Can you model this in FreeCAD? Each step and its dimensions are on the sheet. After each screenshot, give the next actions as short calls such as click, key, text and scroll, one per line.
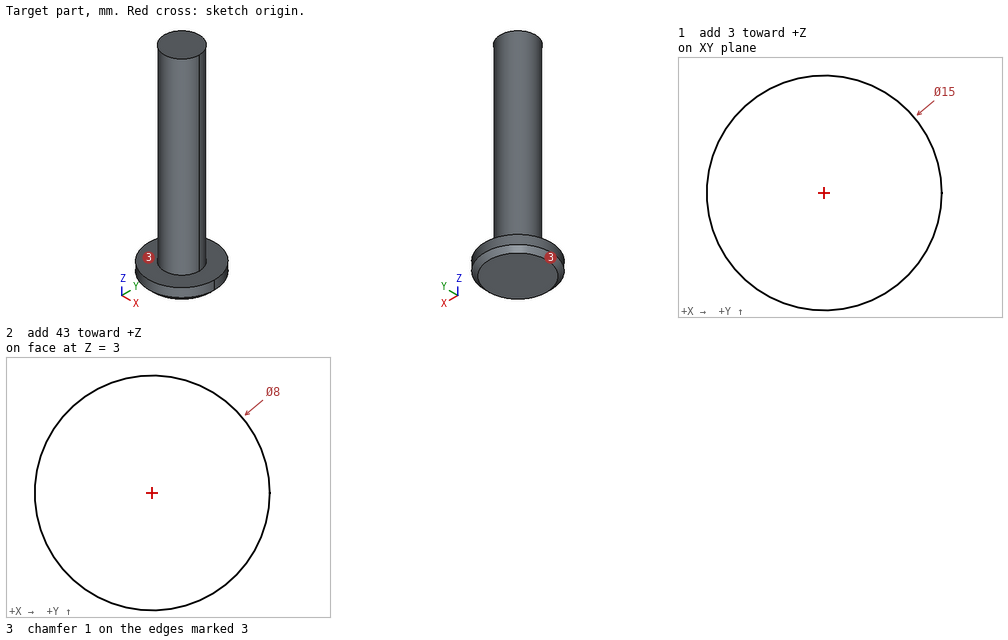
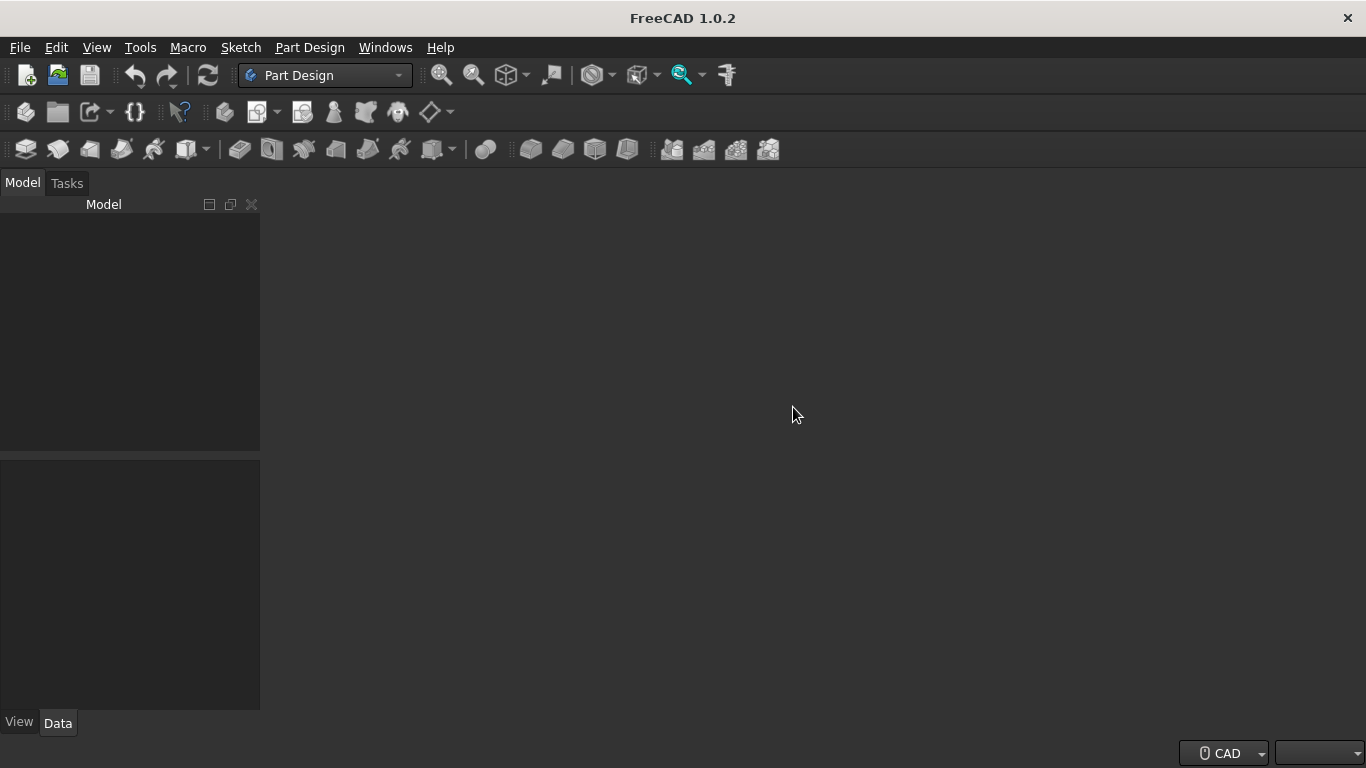
click(26, 76)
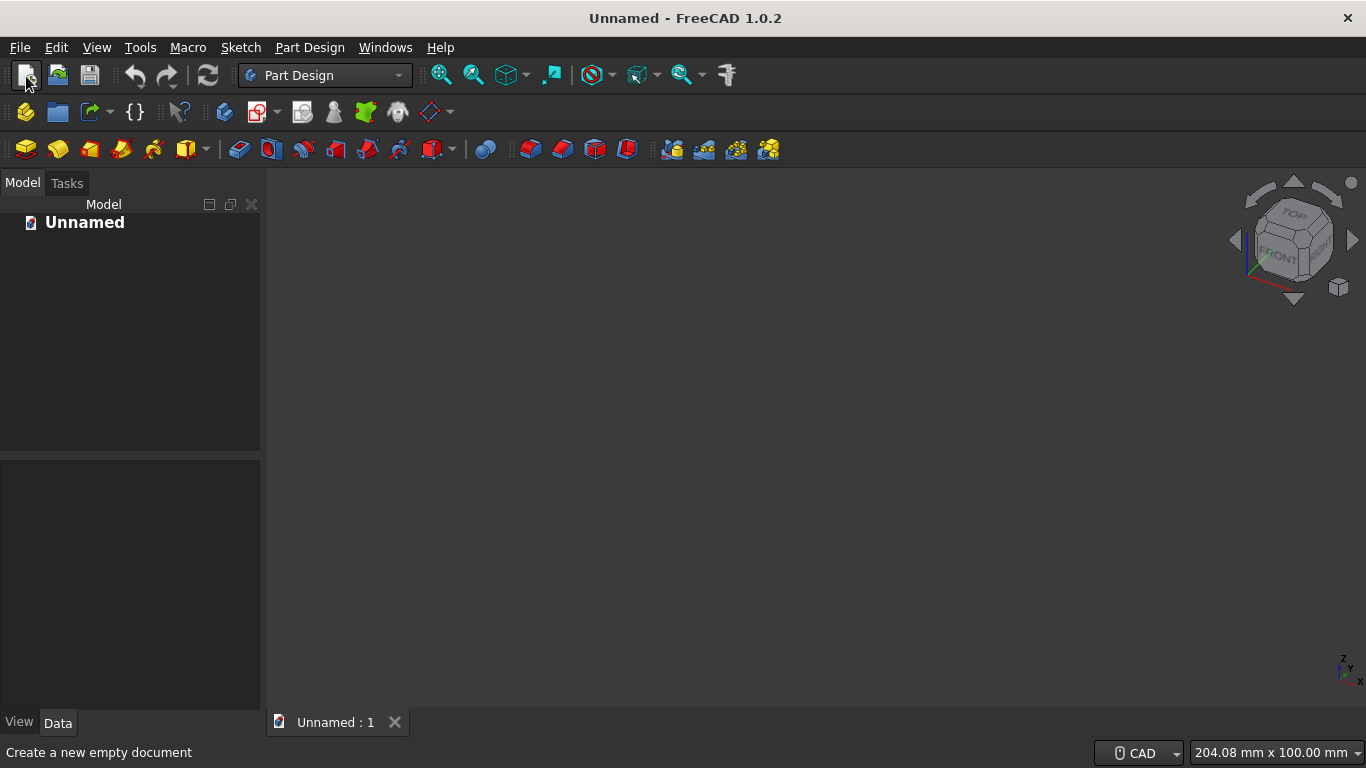
click(258, 112)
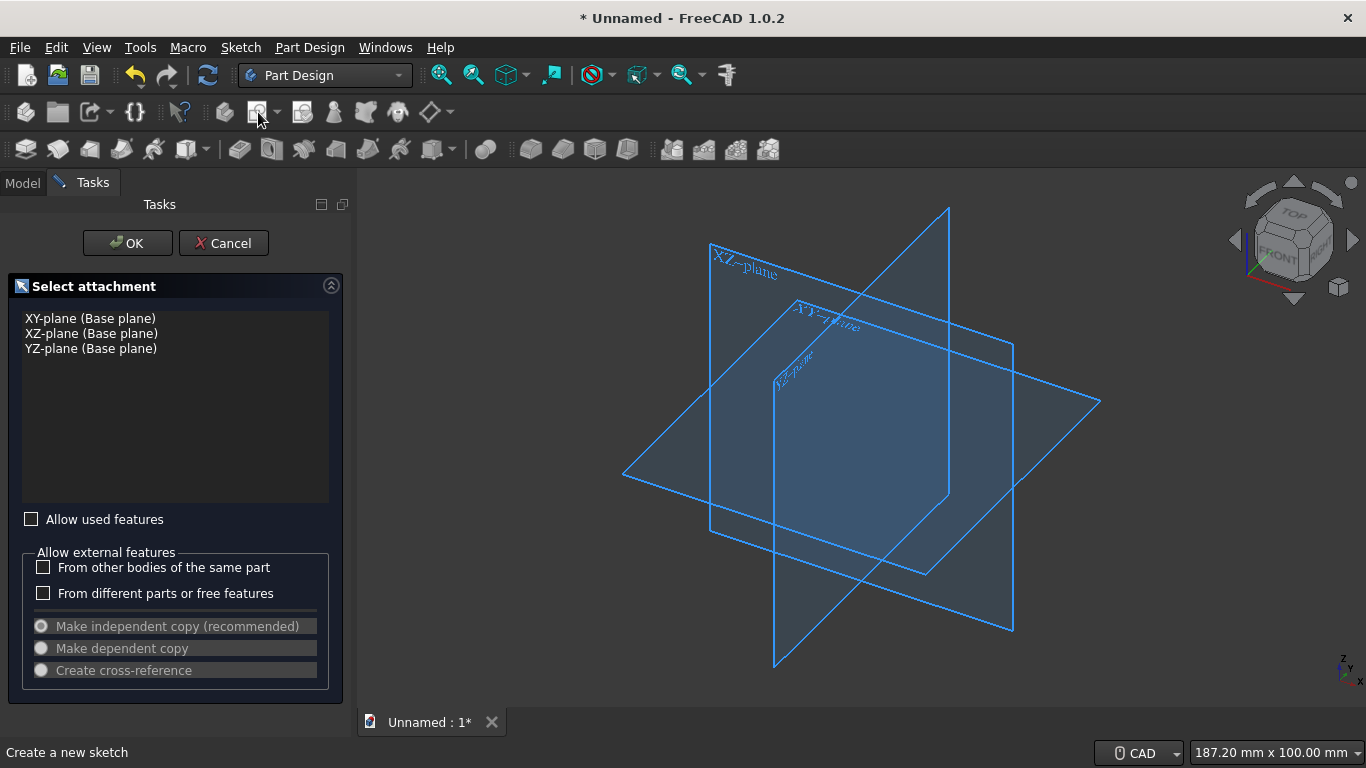
click(82, 318)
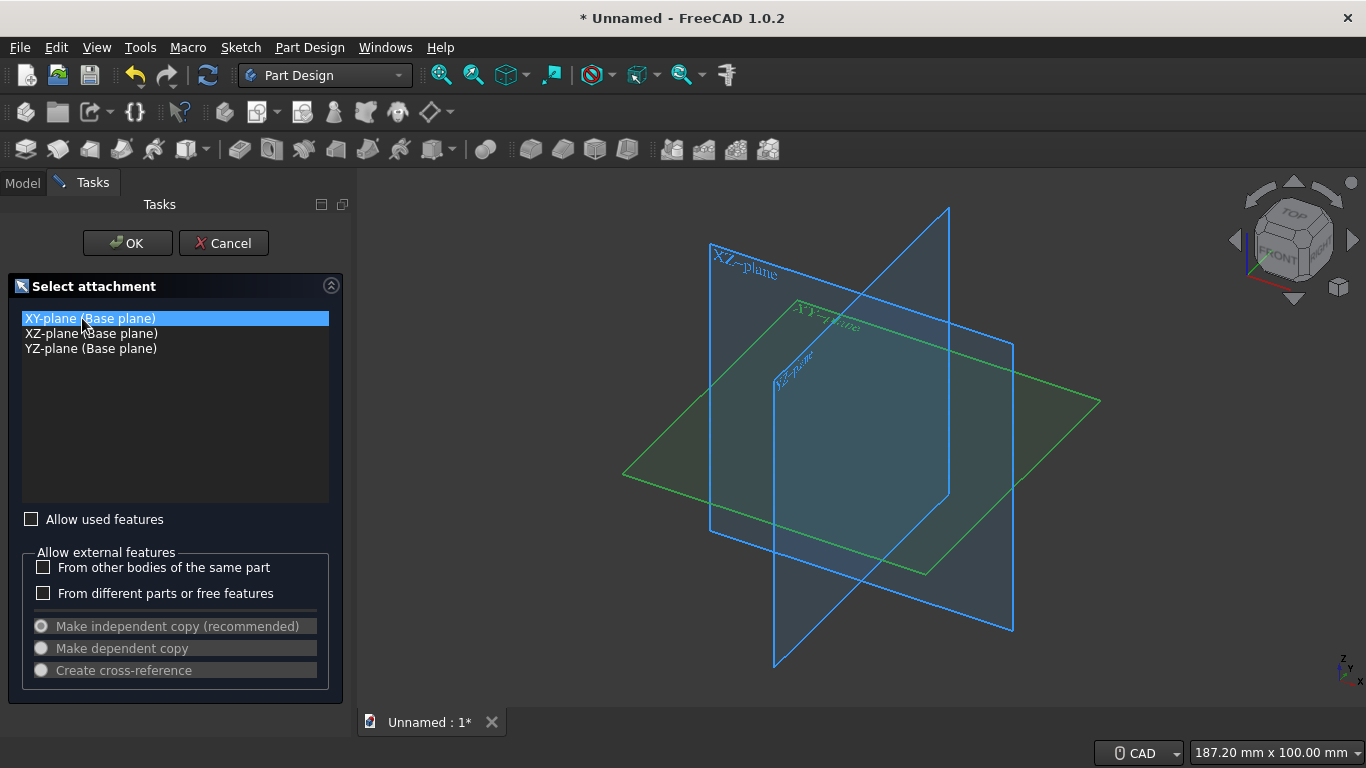
click(128, 243)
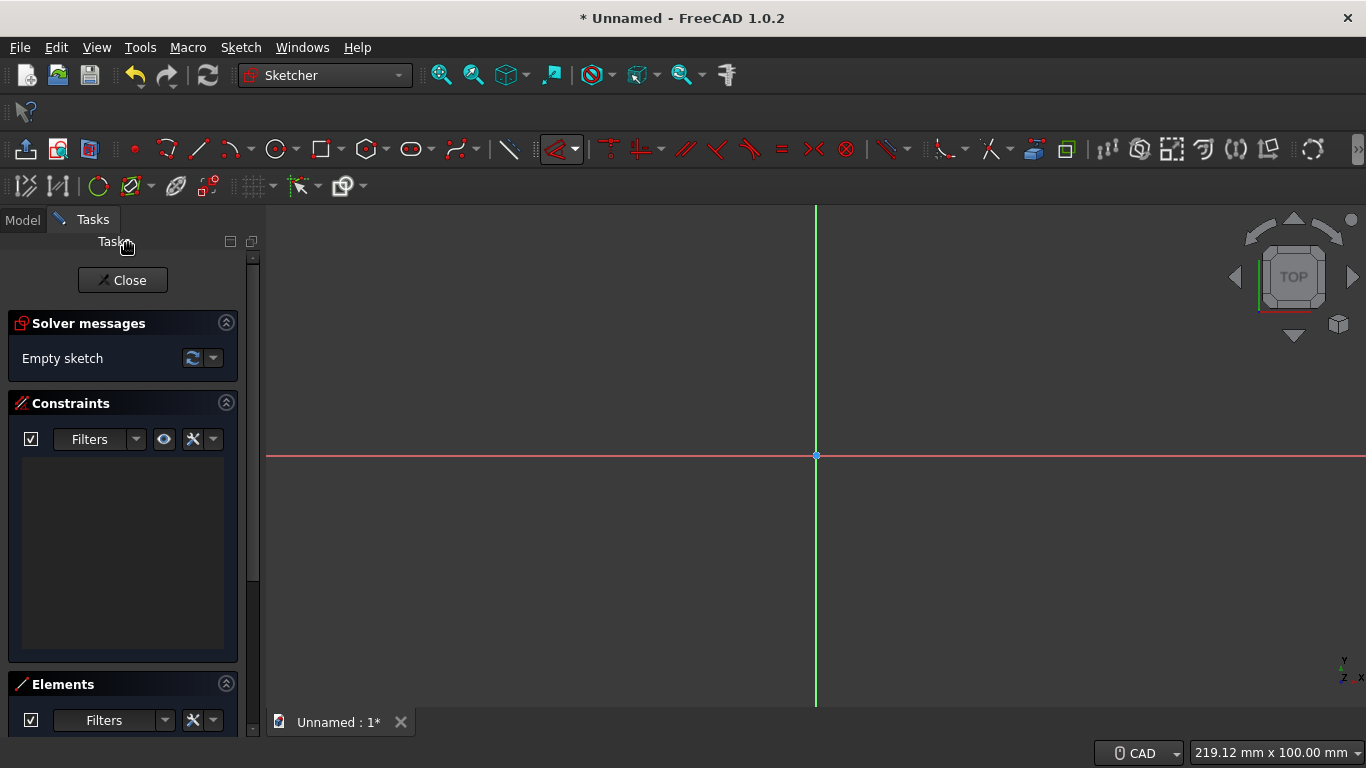
scroll(838, 456, up, 7)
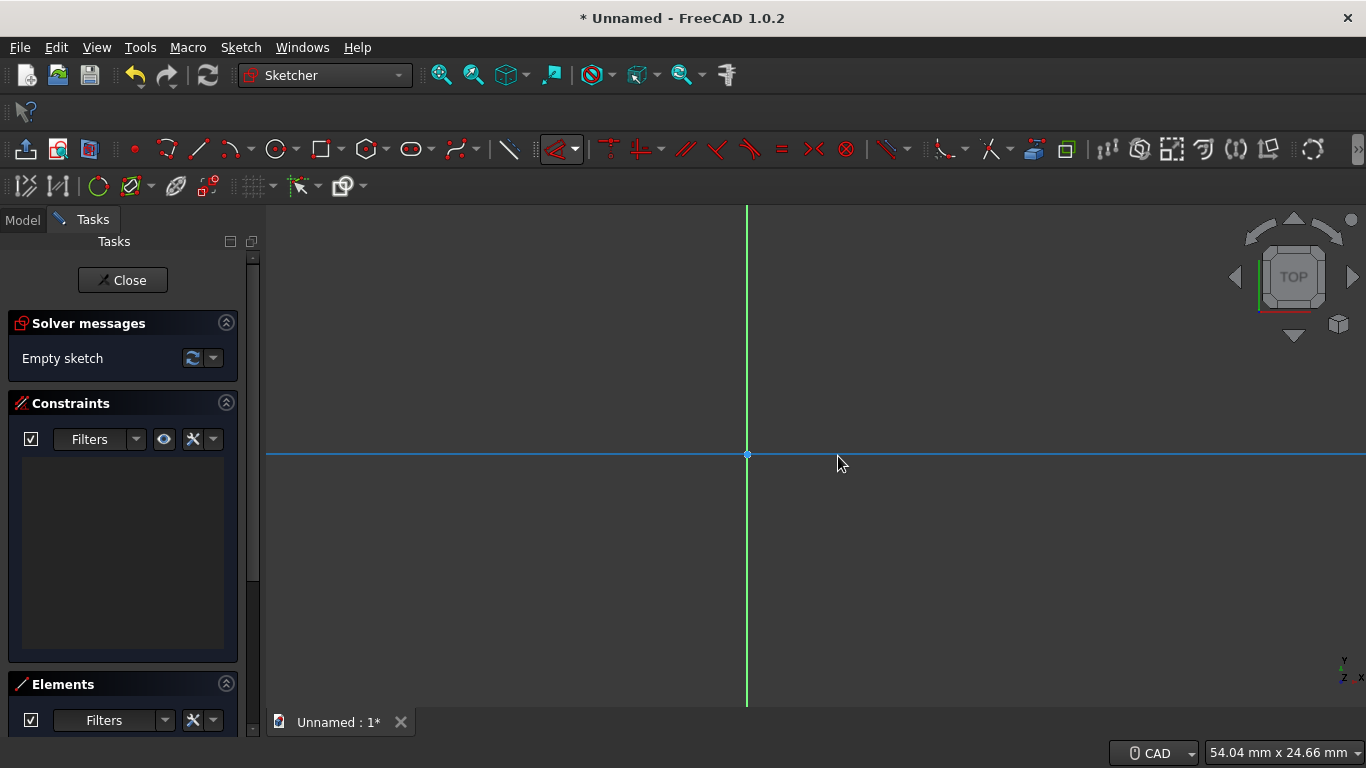
click(276, 150)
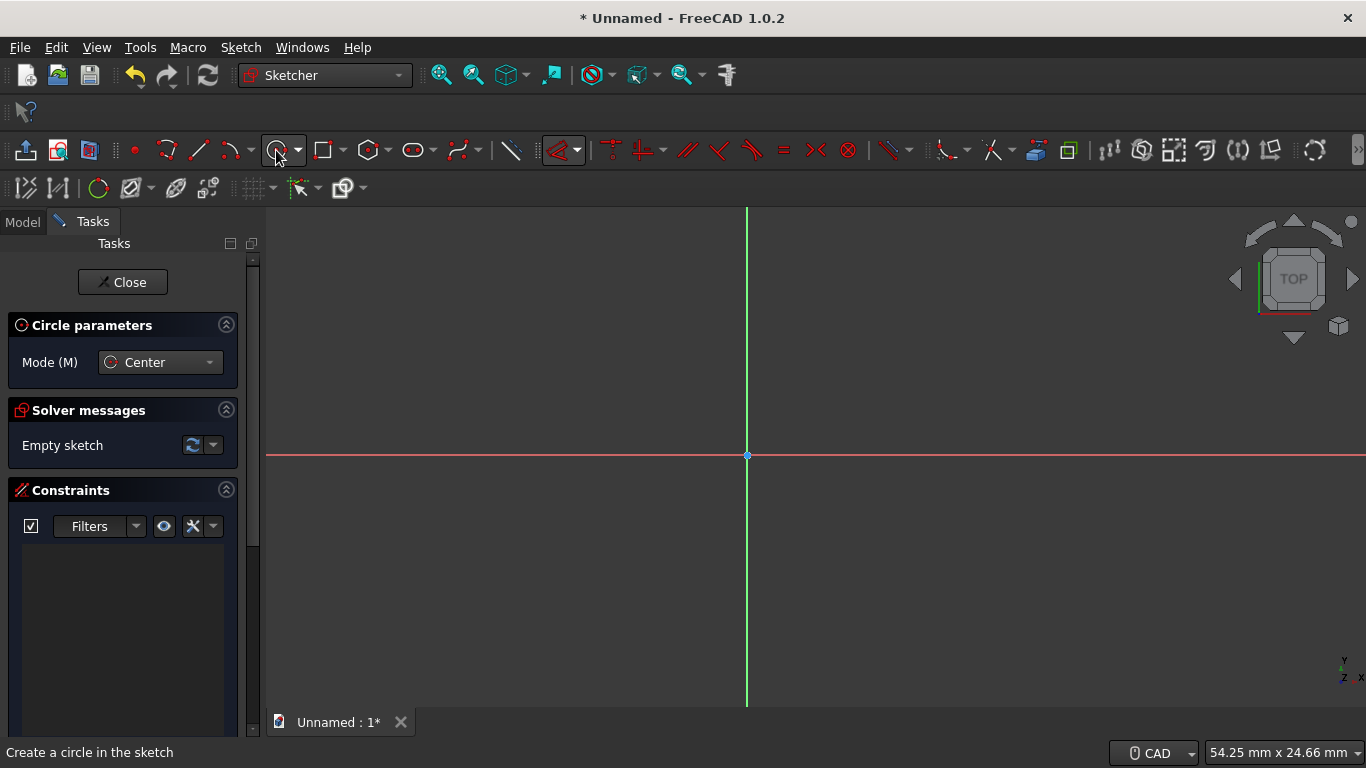
click(747, 455)
click(855, 348)
key(Escape)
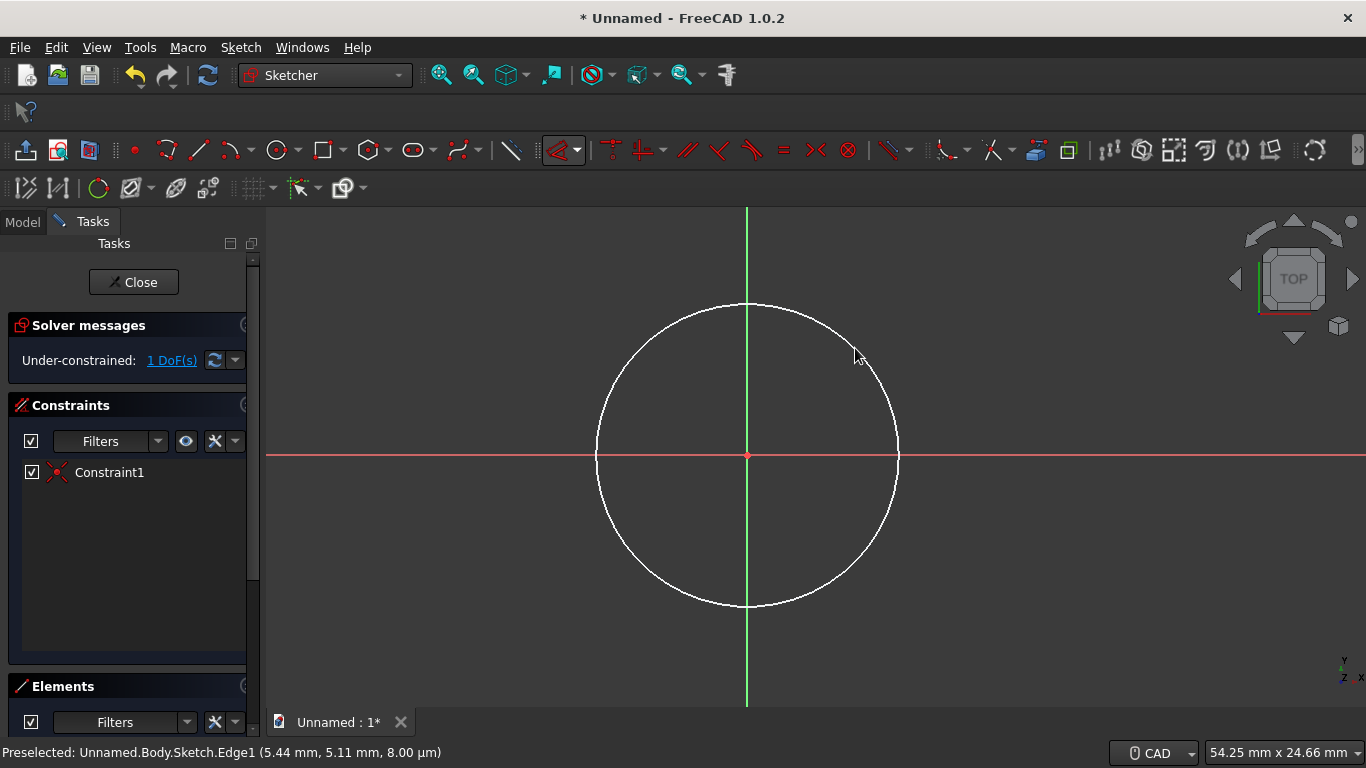
click(558, 150)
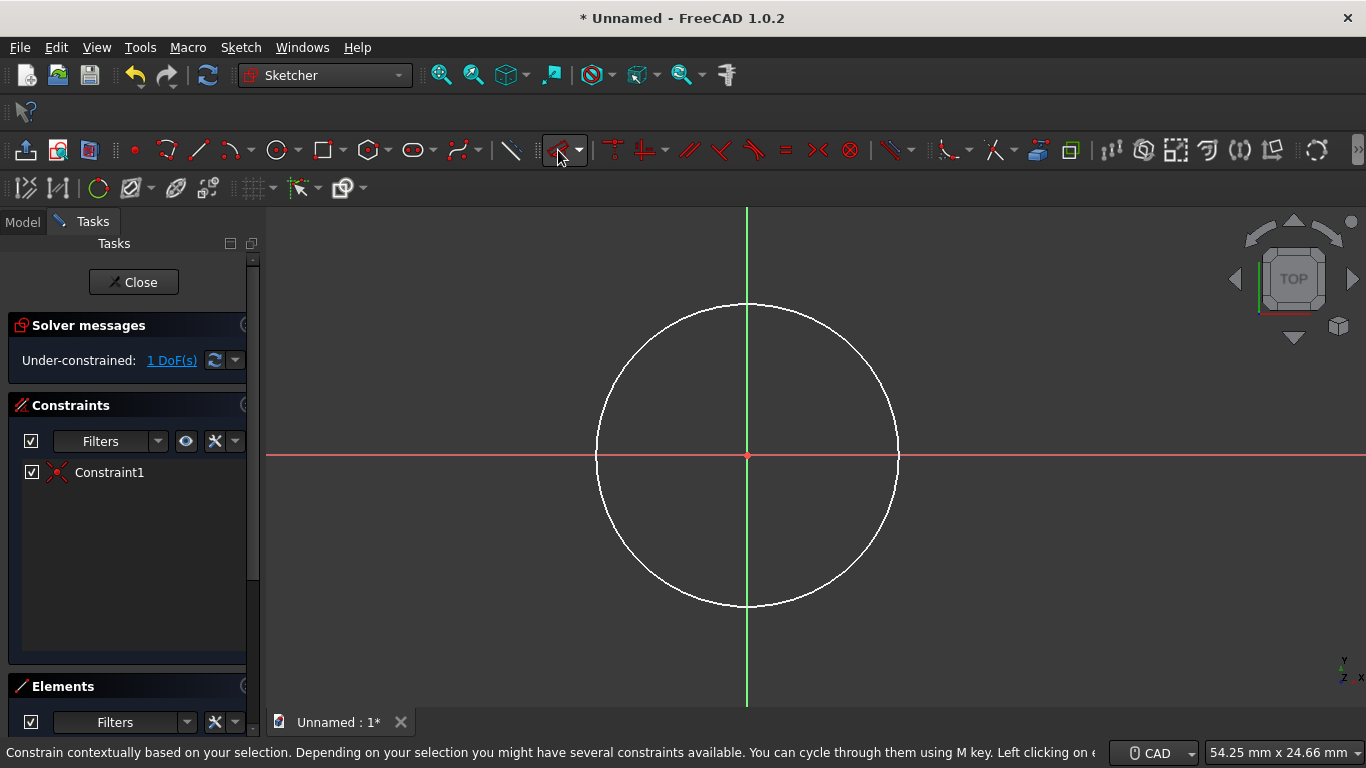
click(854, 348)
click(877, 325)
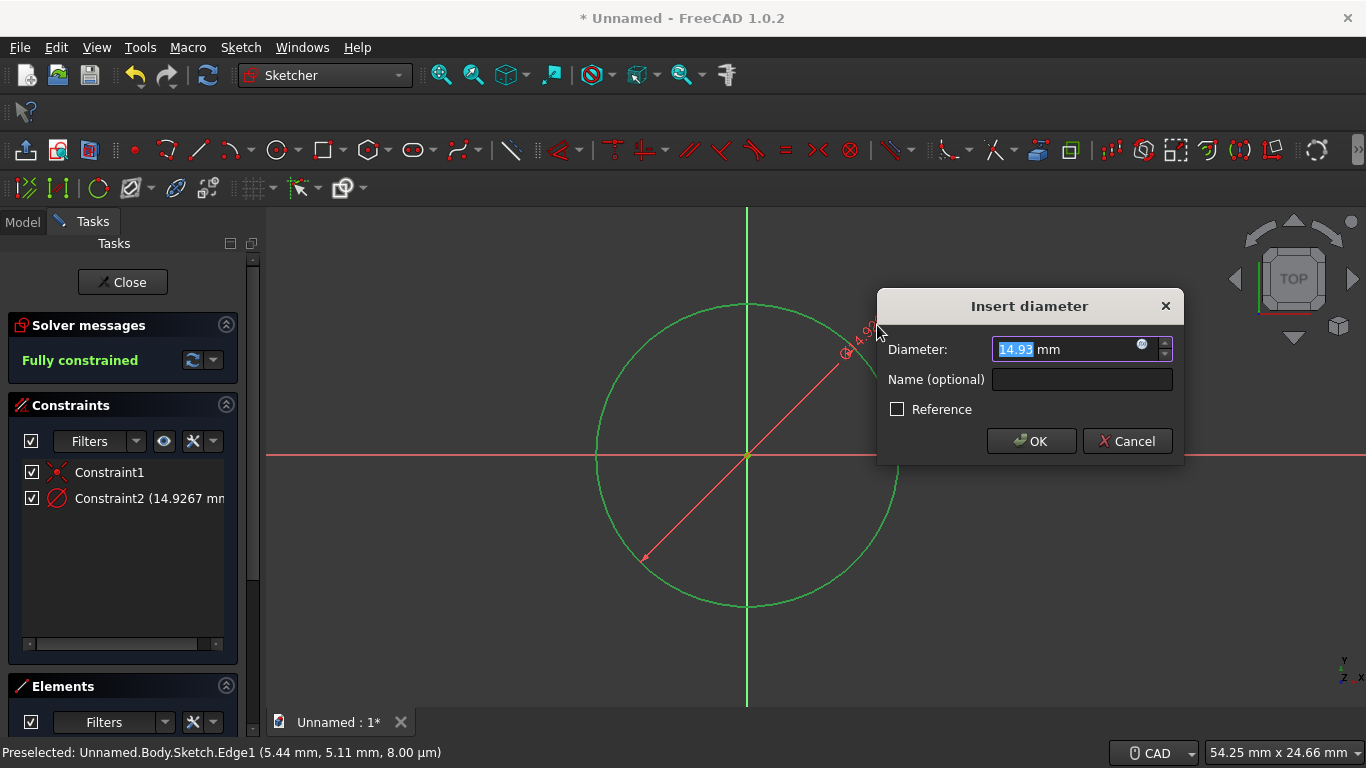
text(15)
key(Return)
key(Escape)